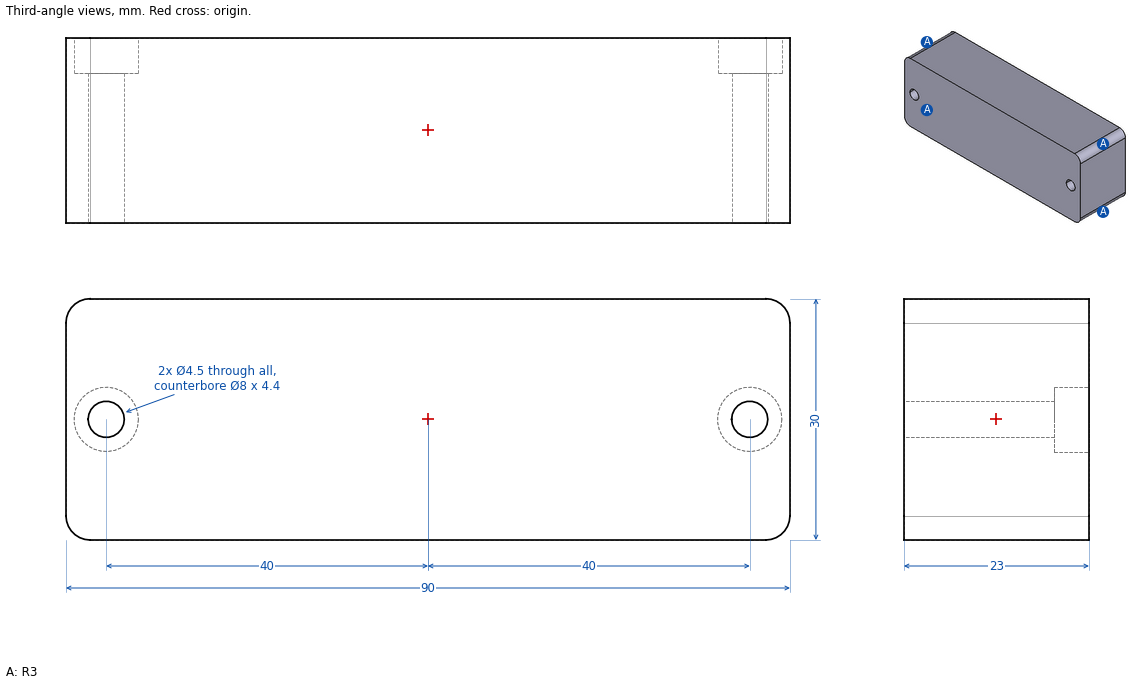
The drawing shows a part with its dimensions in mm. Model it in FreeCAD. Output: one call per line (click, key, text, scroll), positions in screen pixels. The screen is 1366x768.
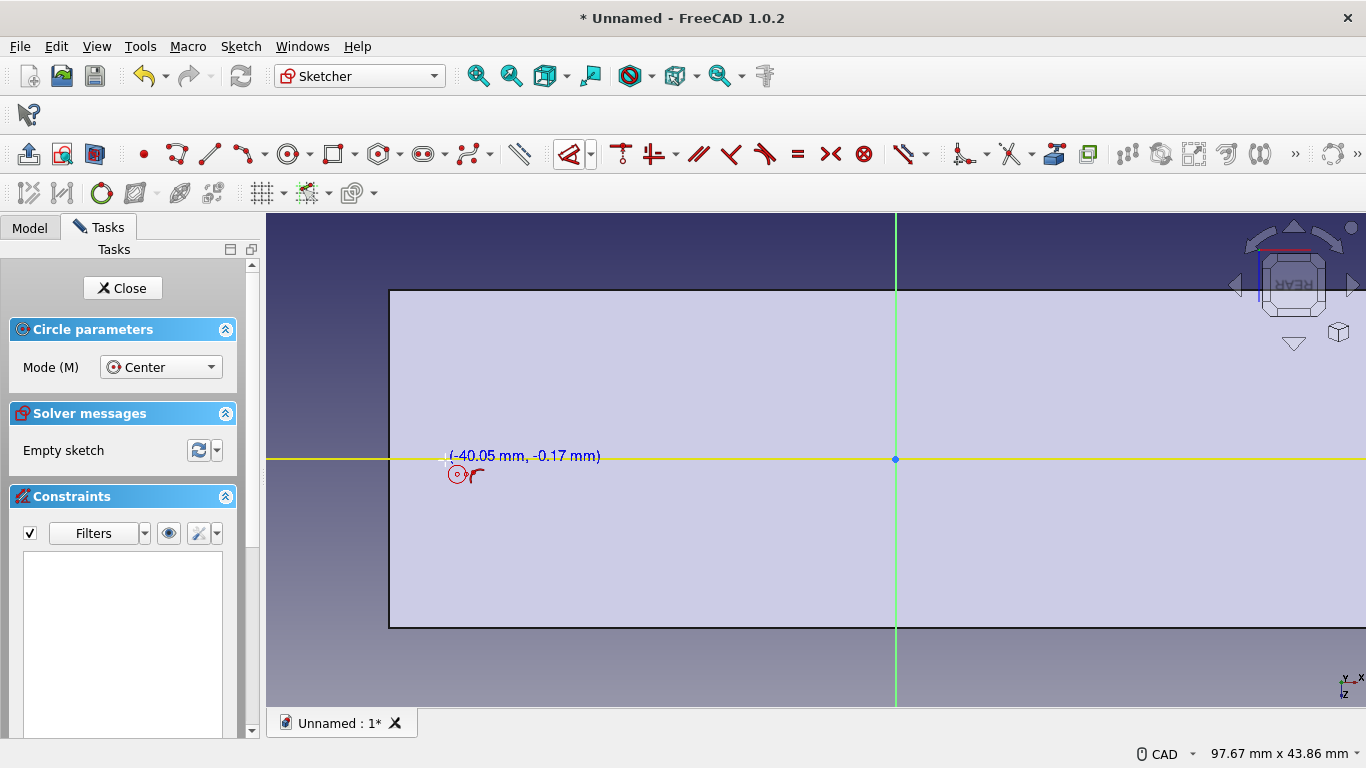
click(445, 459)
move(463, 441)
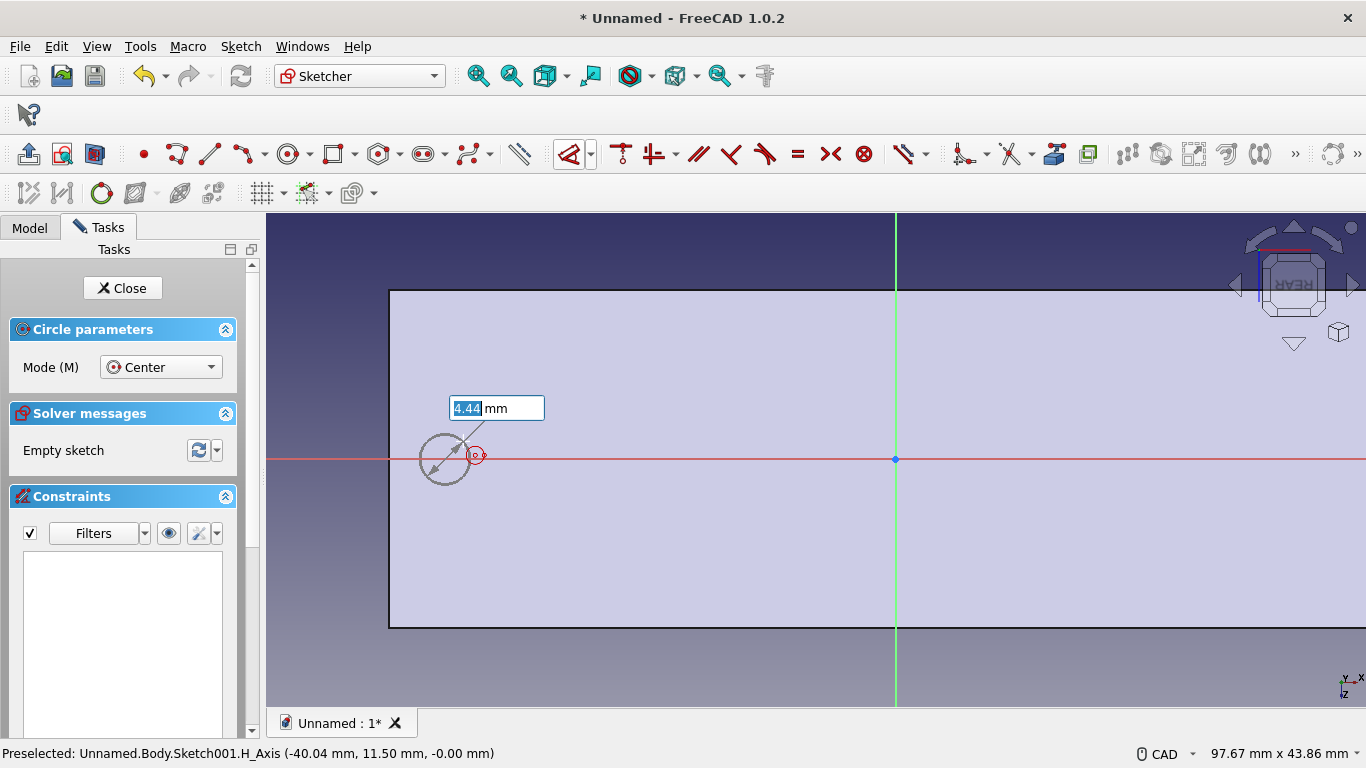
text(4.5)
key(Return)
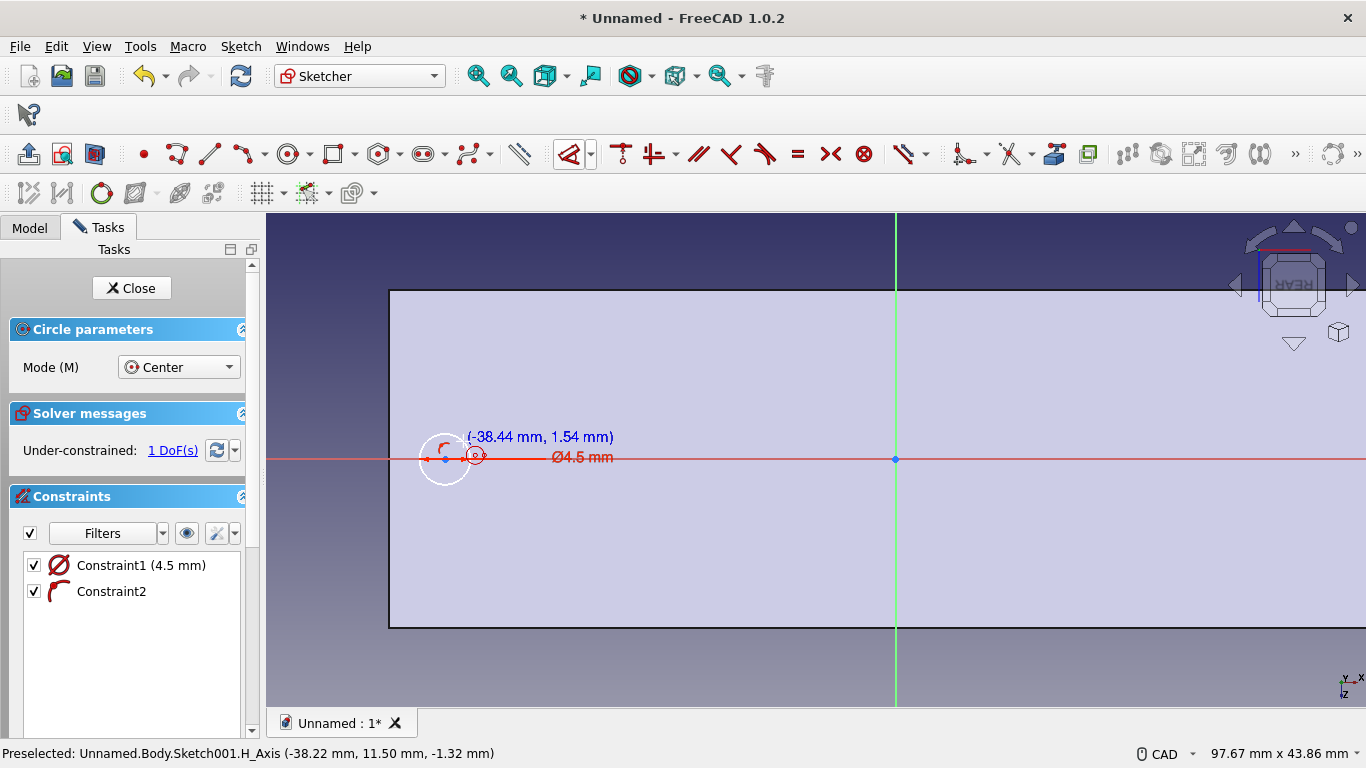
scroll(446, 461, down, 2)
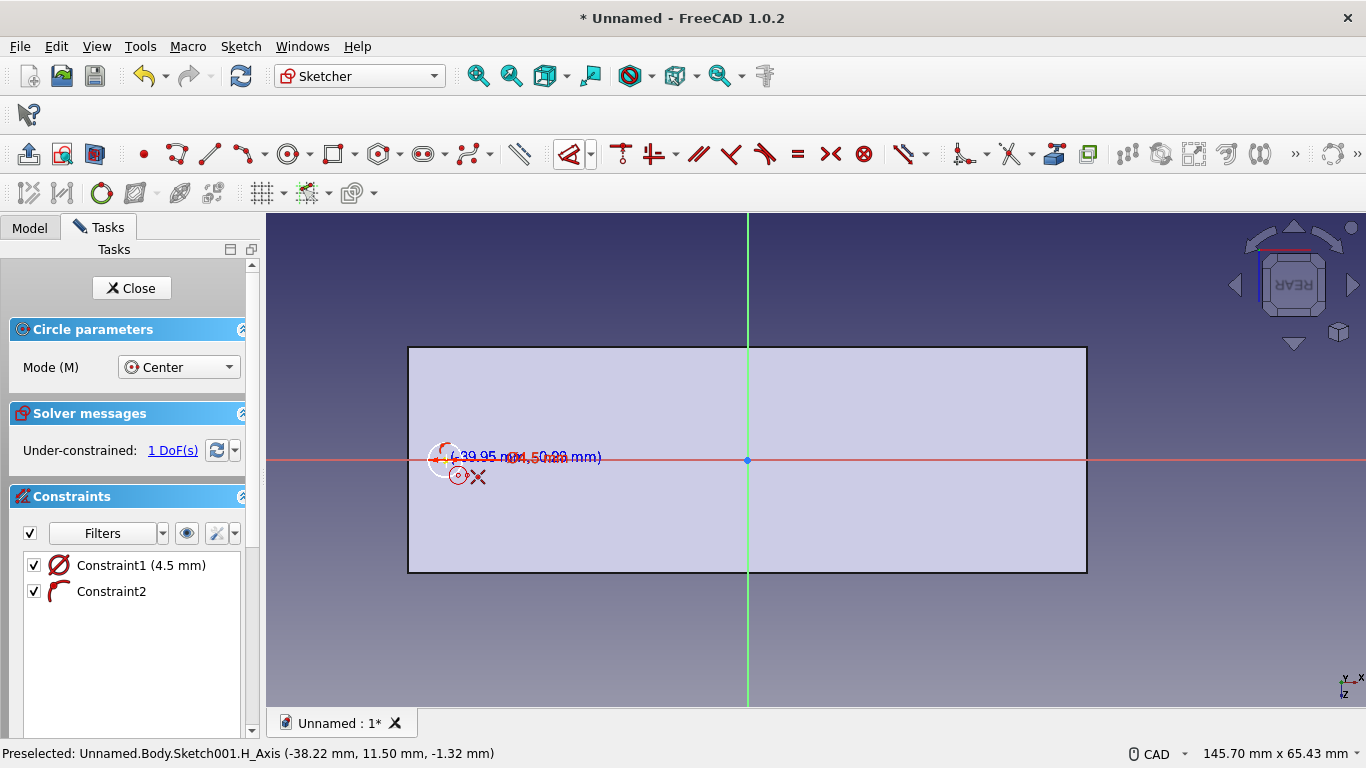
scroll(1050, 460, up, 2)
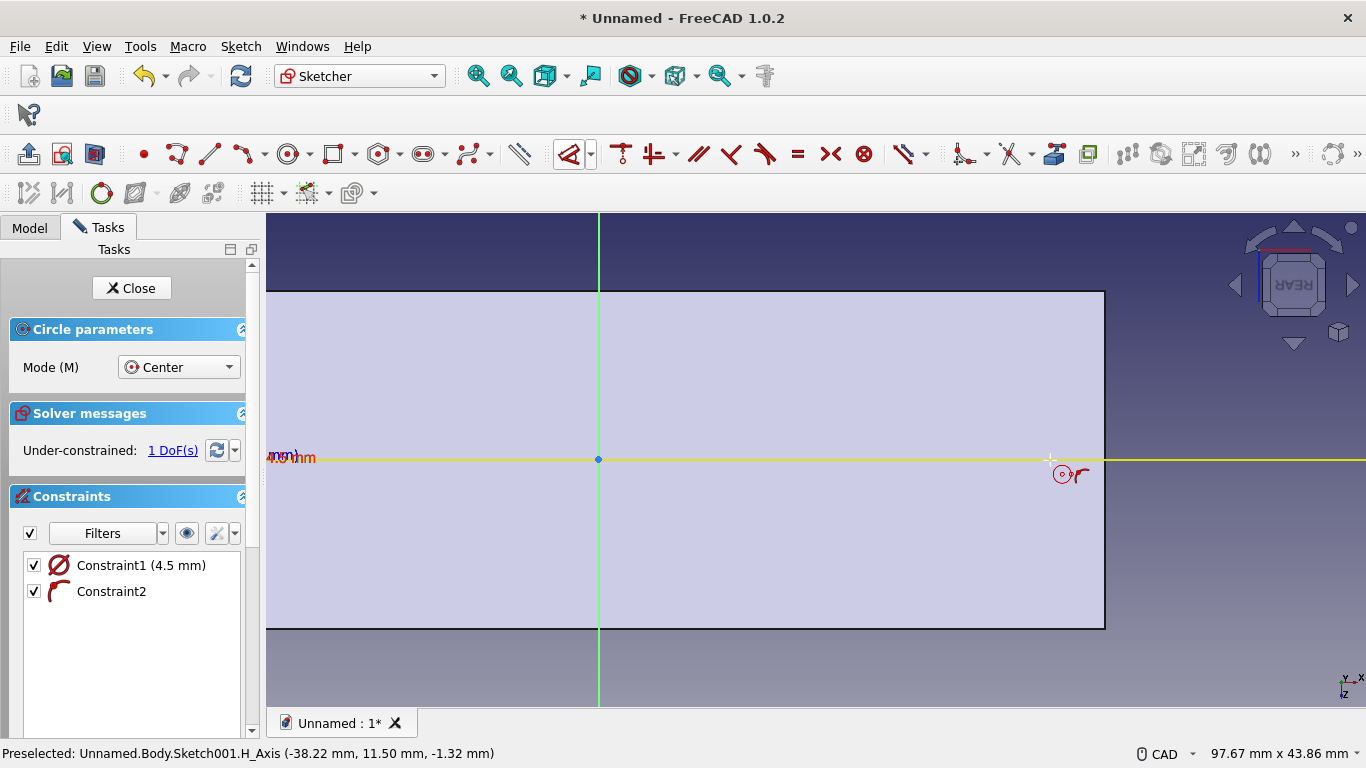
click(1049, 460)
move(1067, 442)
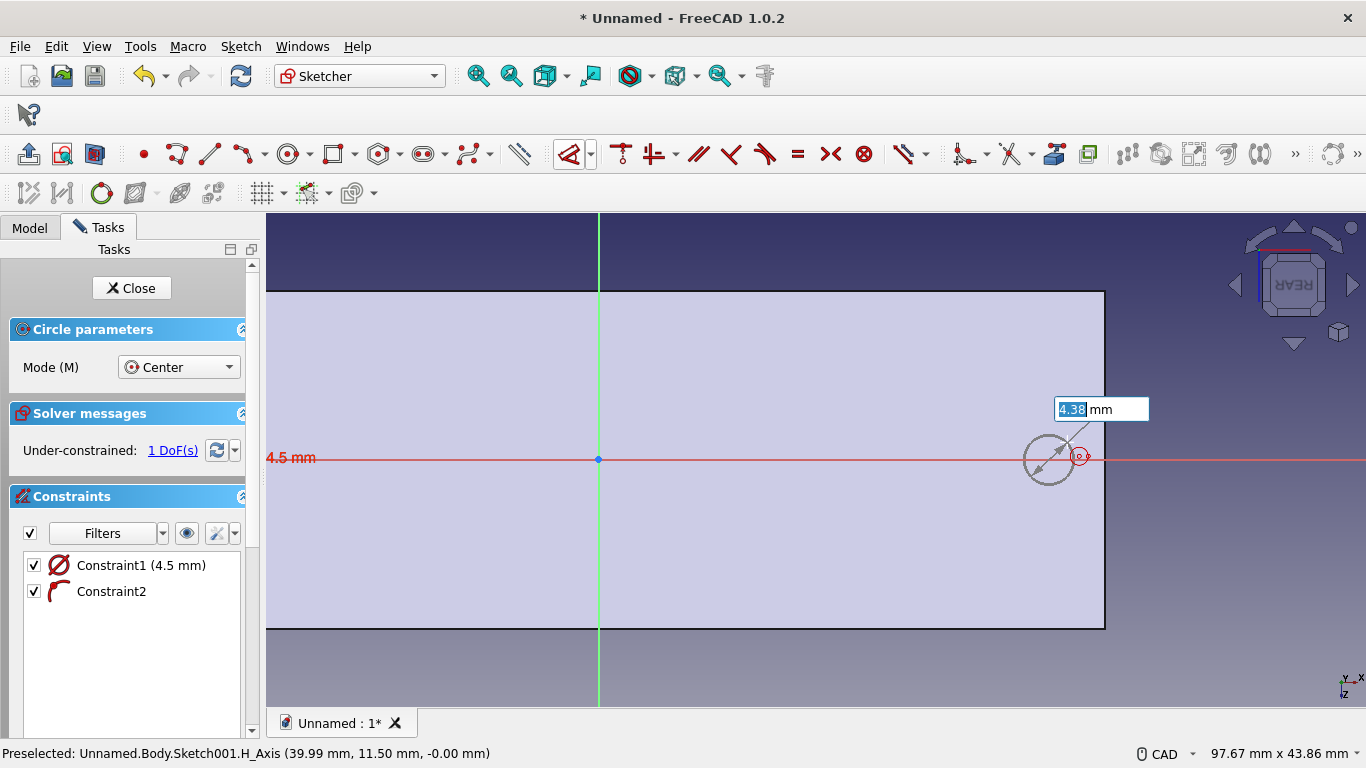
text(4.5)
key(Return)
key(Escape)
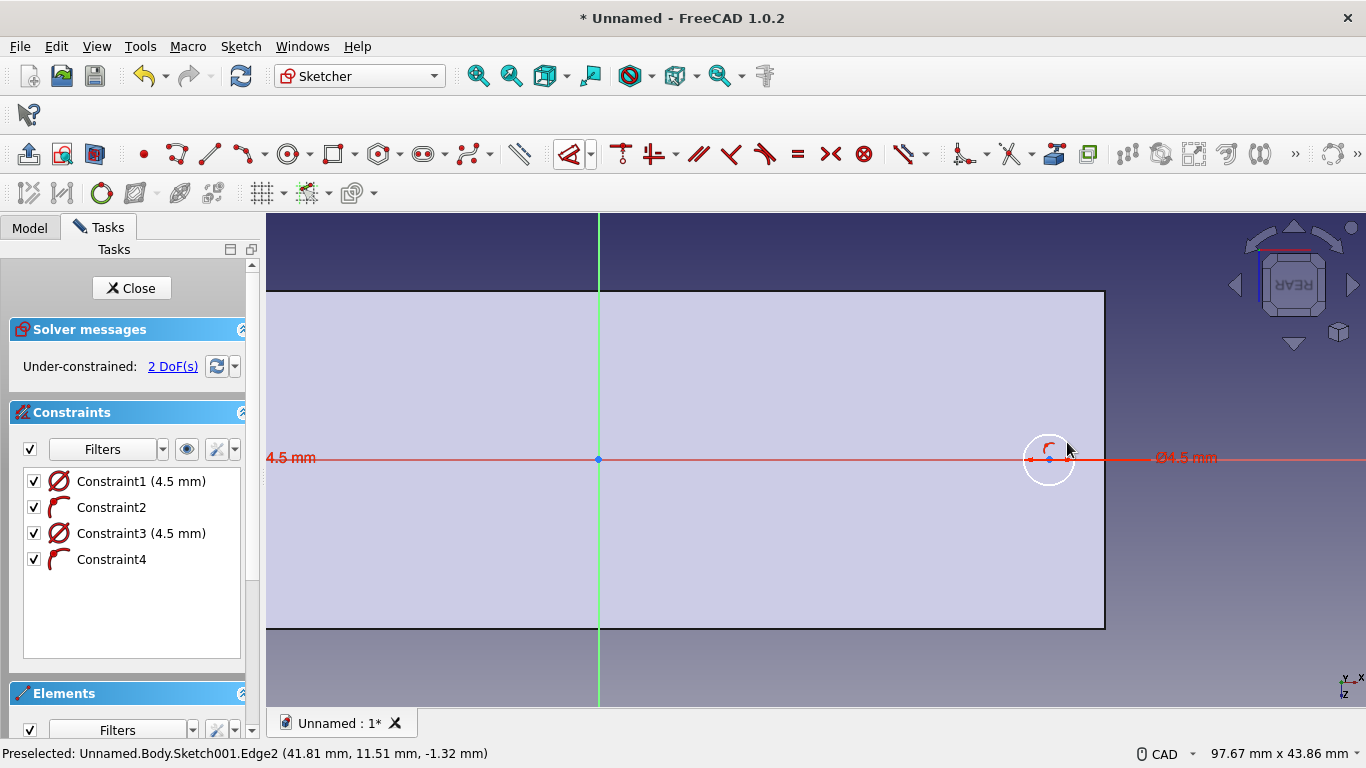
scroll(1050, 460, down, 2)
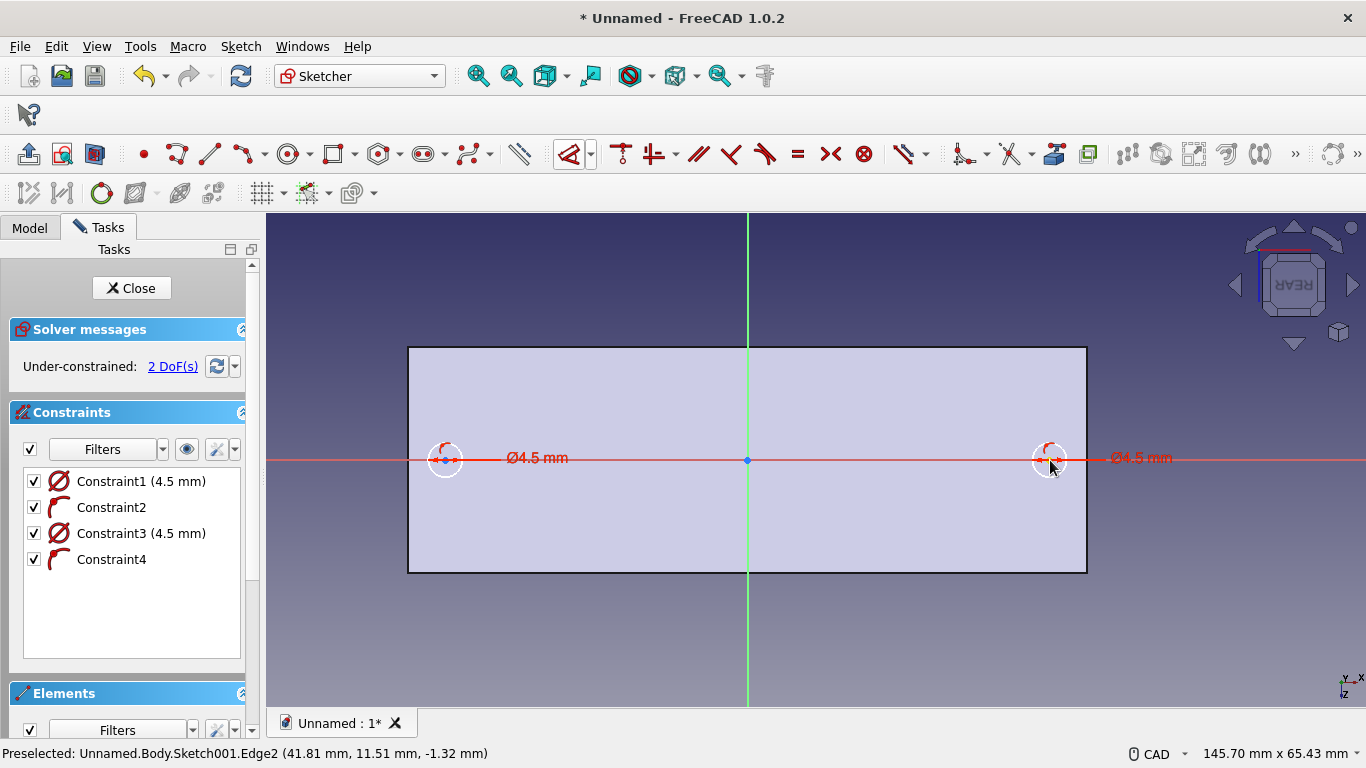
click(445, 460)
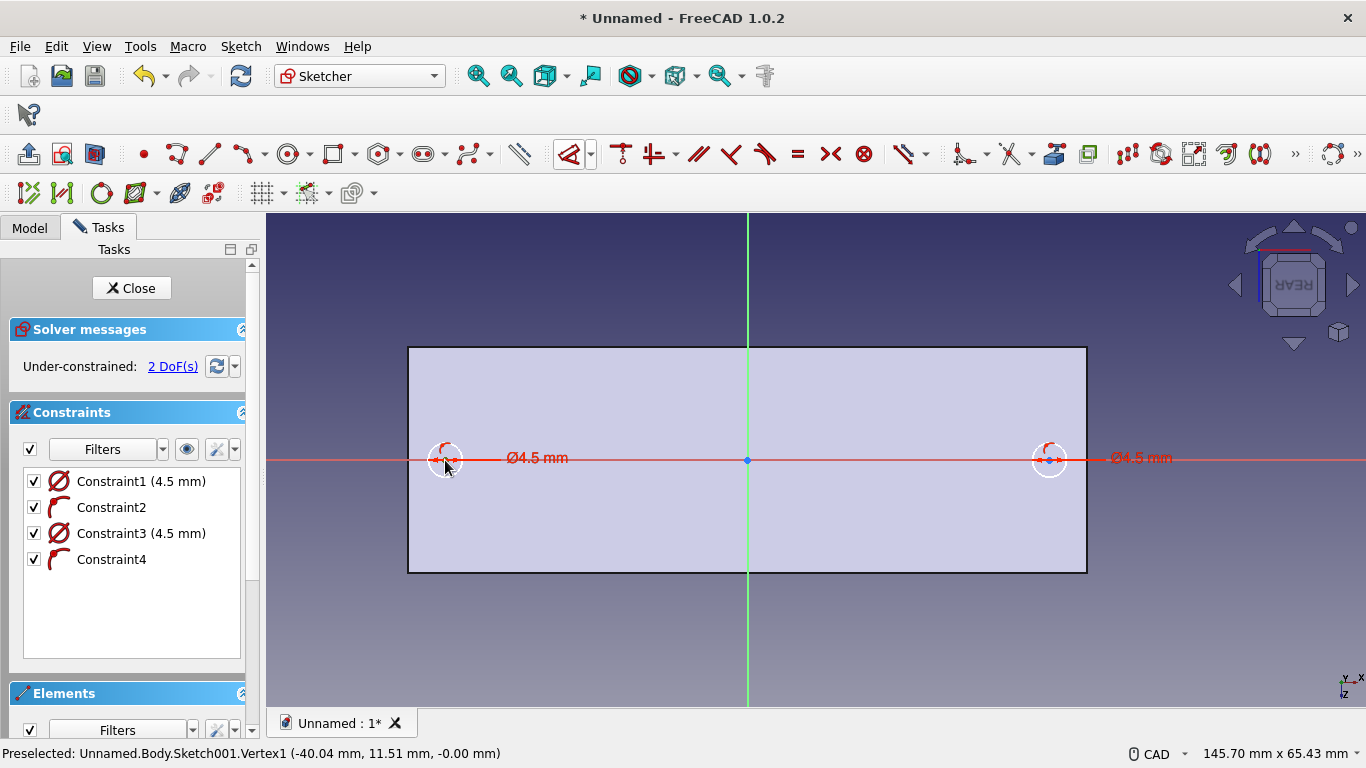
key(l)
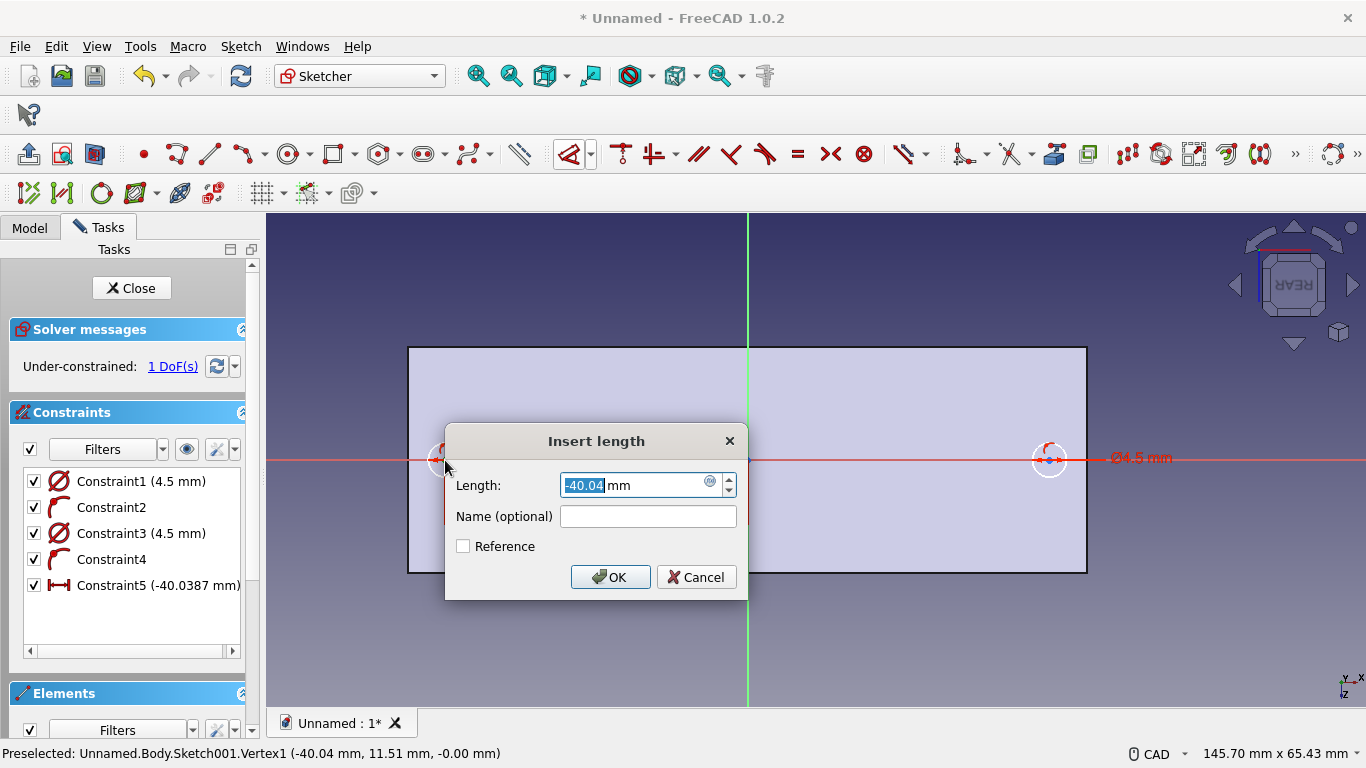
text(-40)
key(Return)